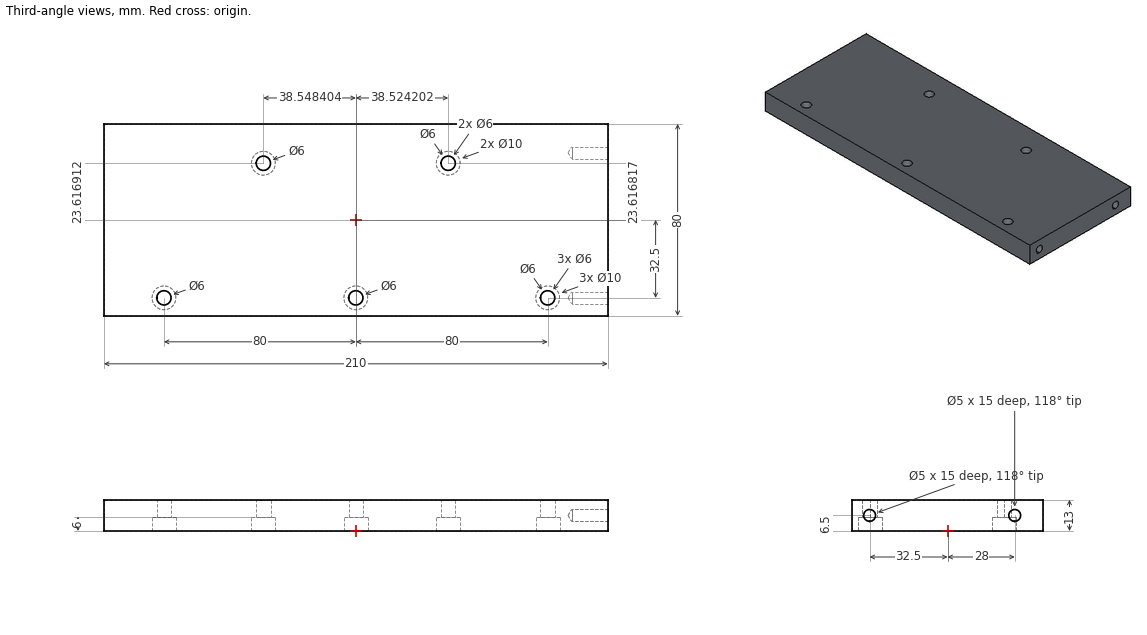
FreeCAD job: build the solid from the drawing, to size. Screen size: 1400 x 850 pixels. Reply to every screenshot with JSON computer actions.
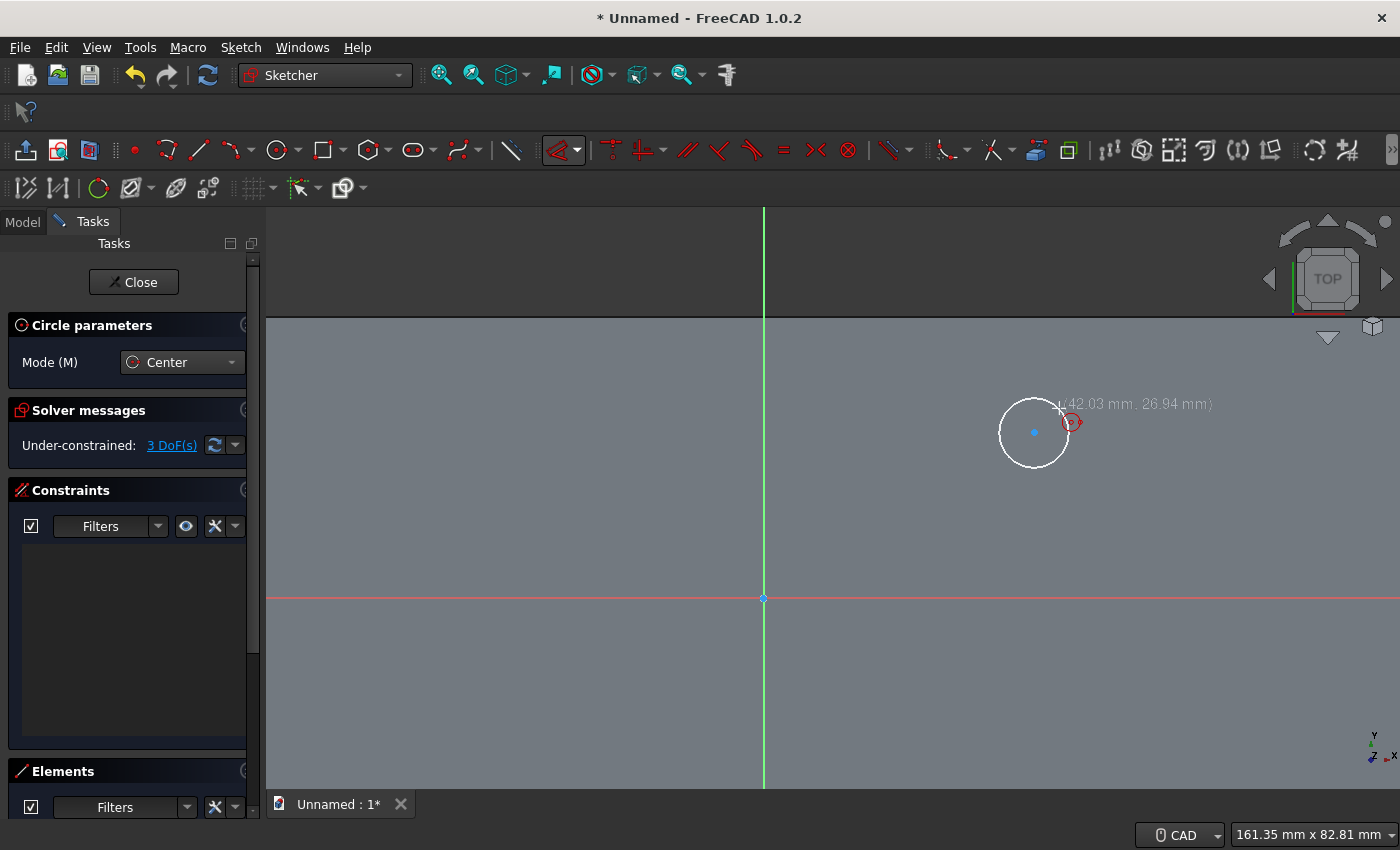
{"action": "left_click", "coordinate": [493, 432]}
{"action": "left_click", "coordinate": [518, 408]}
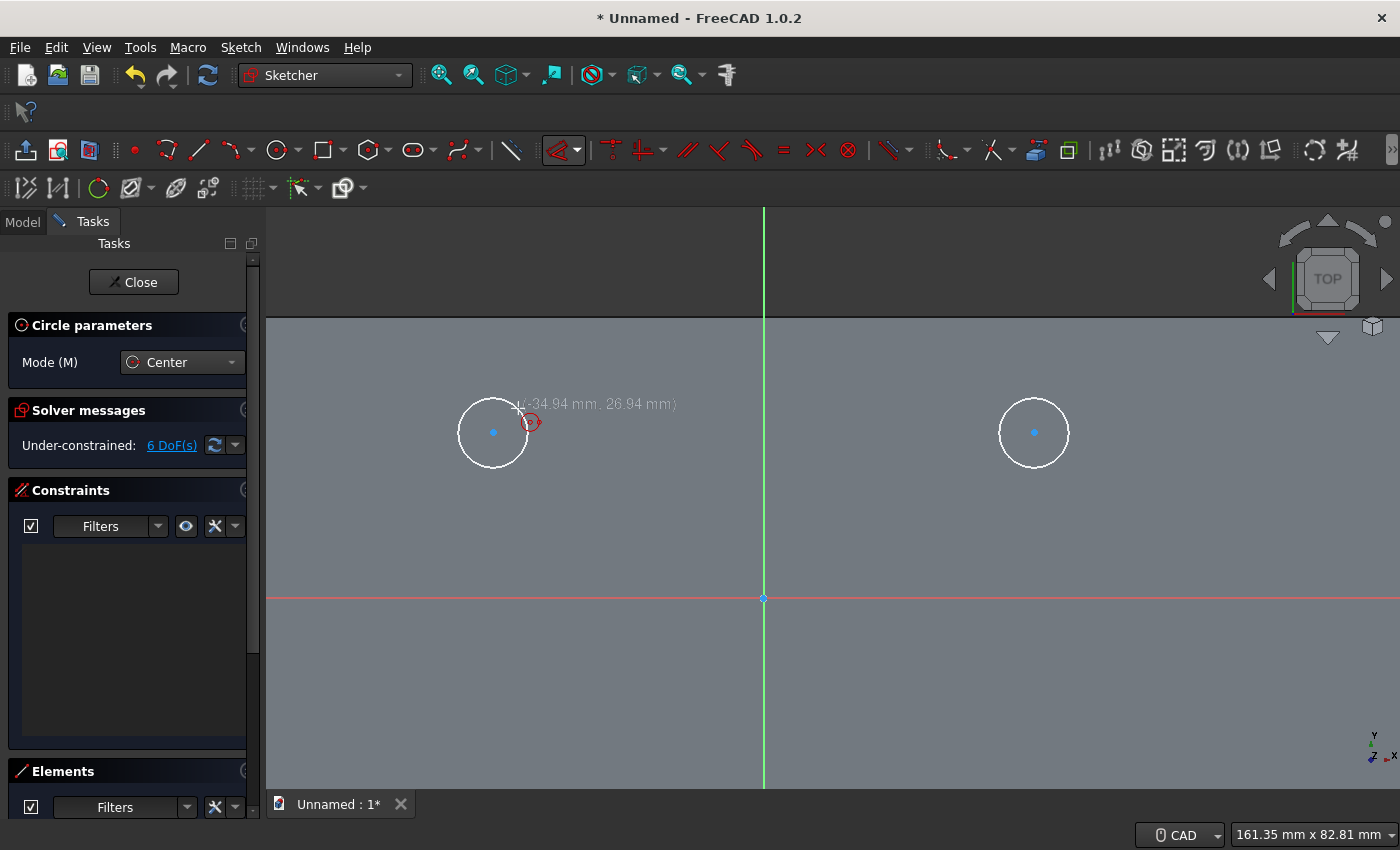
{"action": "left_click", "coordinate": [1034, 433]}
{"action": "left_click", "coordinate": [1049, 417]}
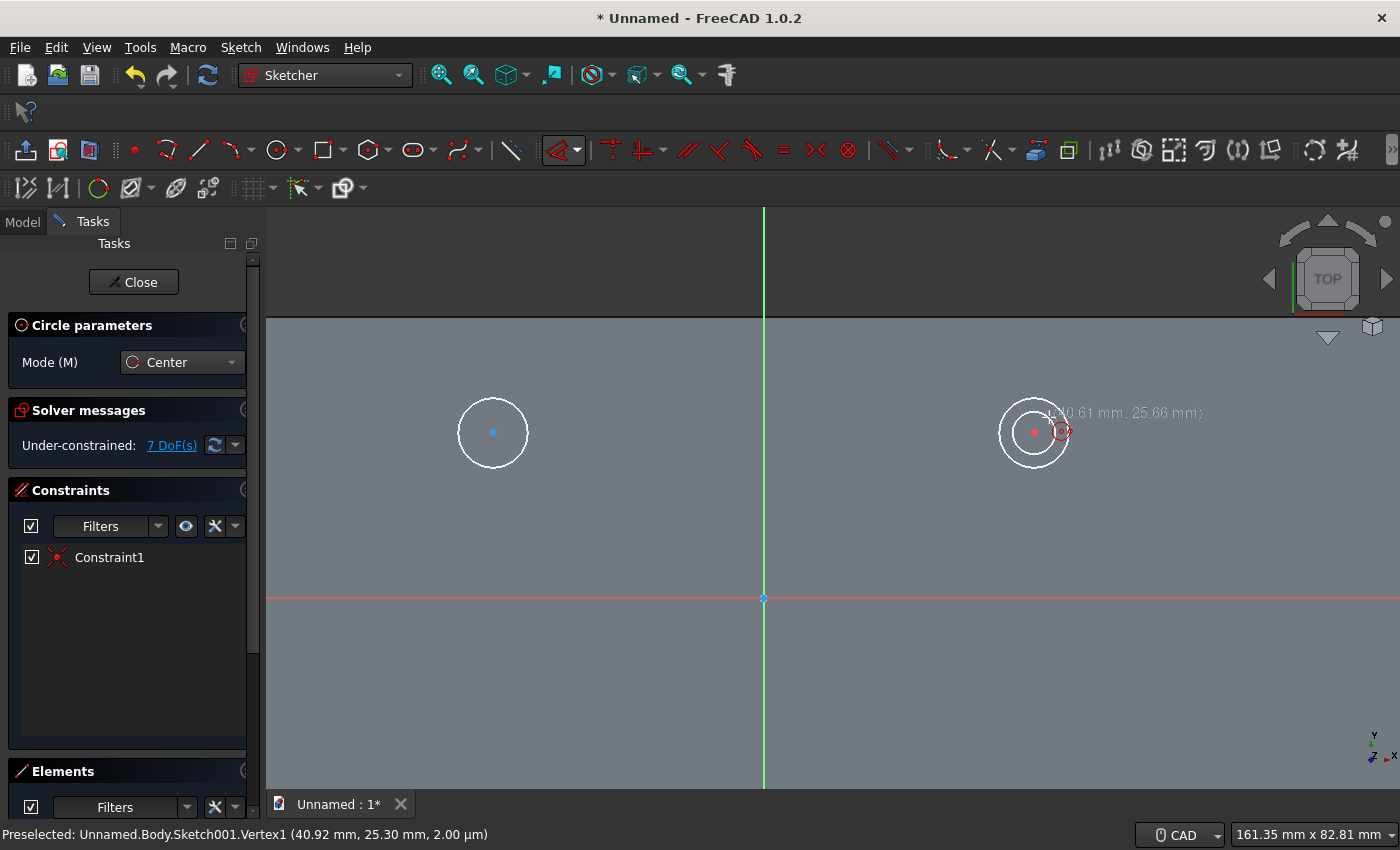
{"action": "left_click", "coordinate": [493, 433]}
{"action": "left_click", "coordinate": [508, 417]}
{"action": "key", "text": "Escape"}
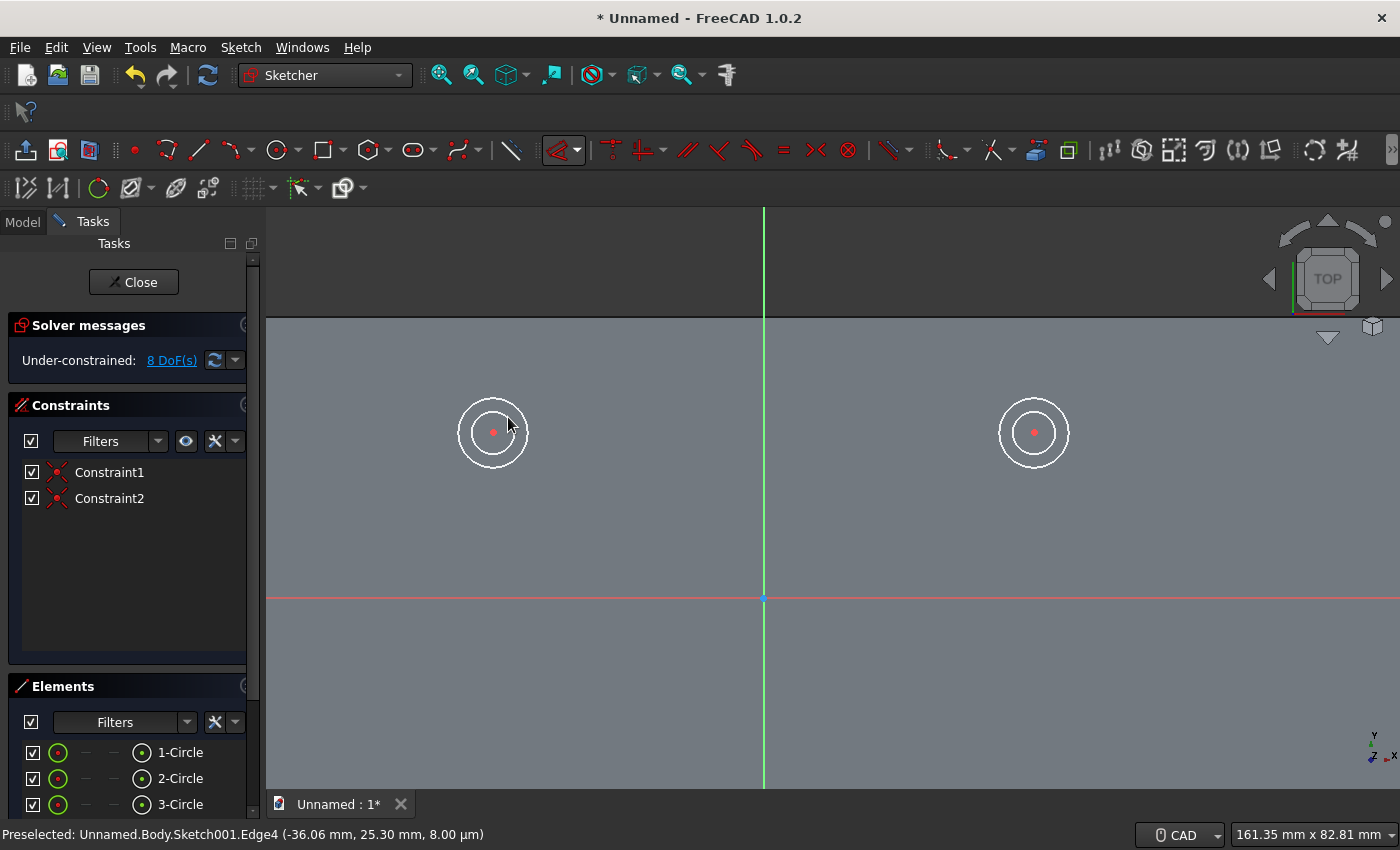
{"action": "left_click", "coordinate": [1058, 408]}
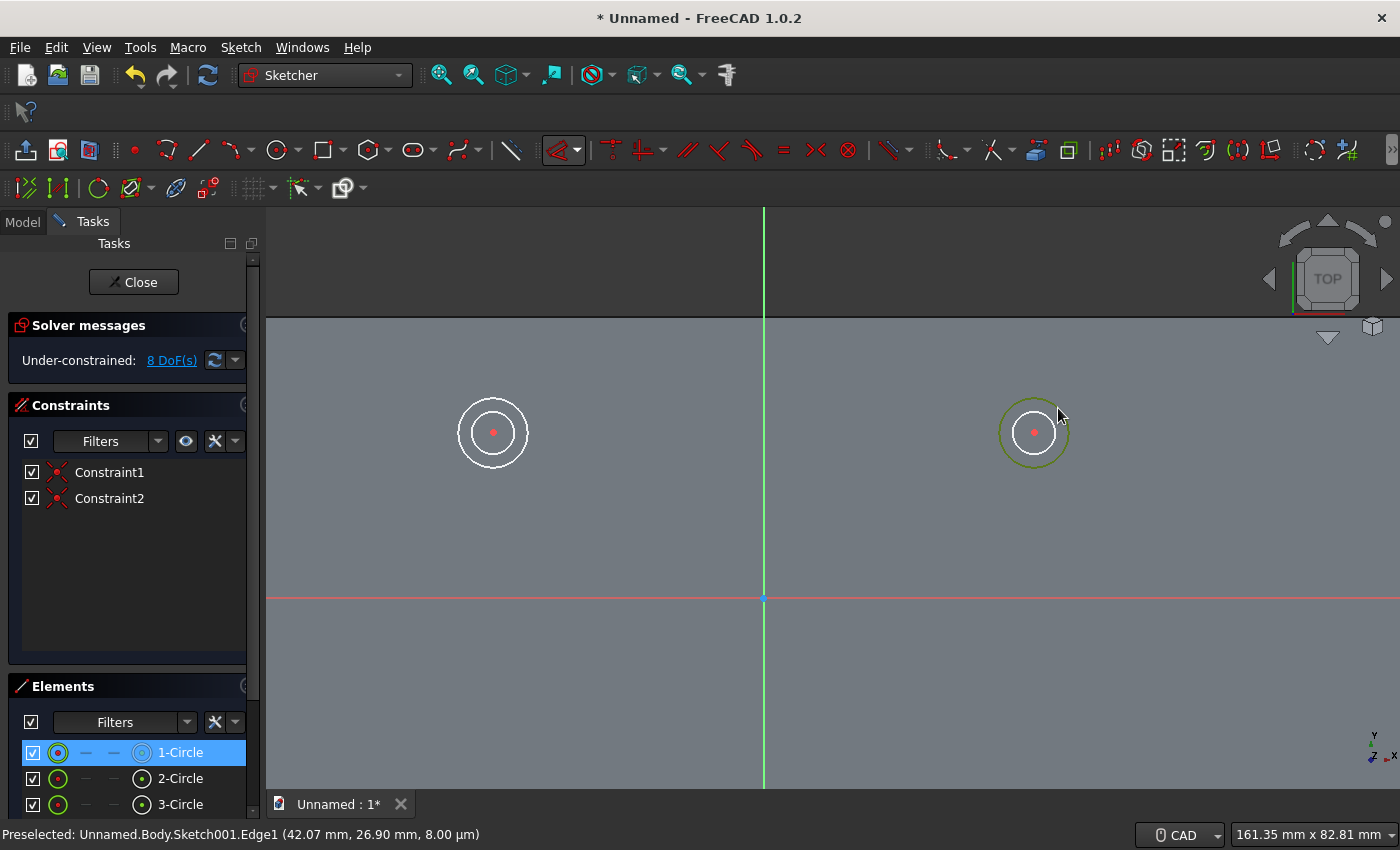
{"action": "left_click", "coordinate": [517, 408]}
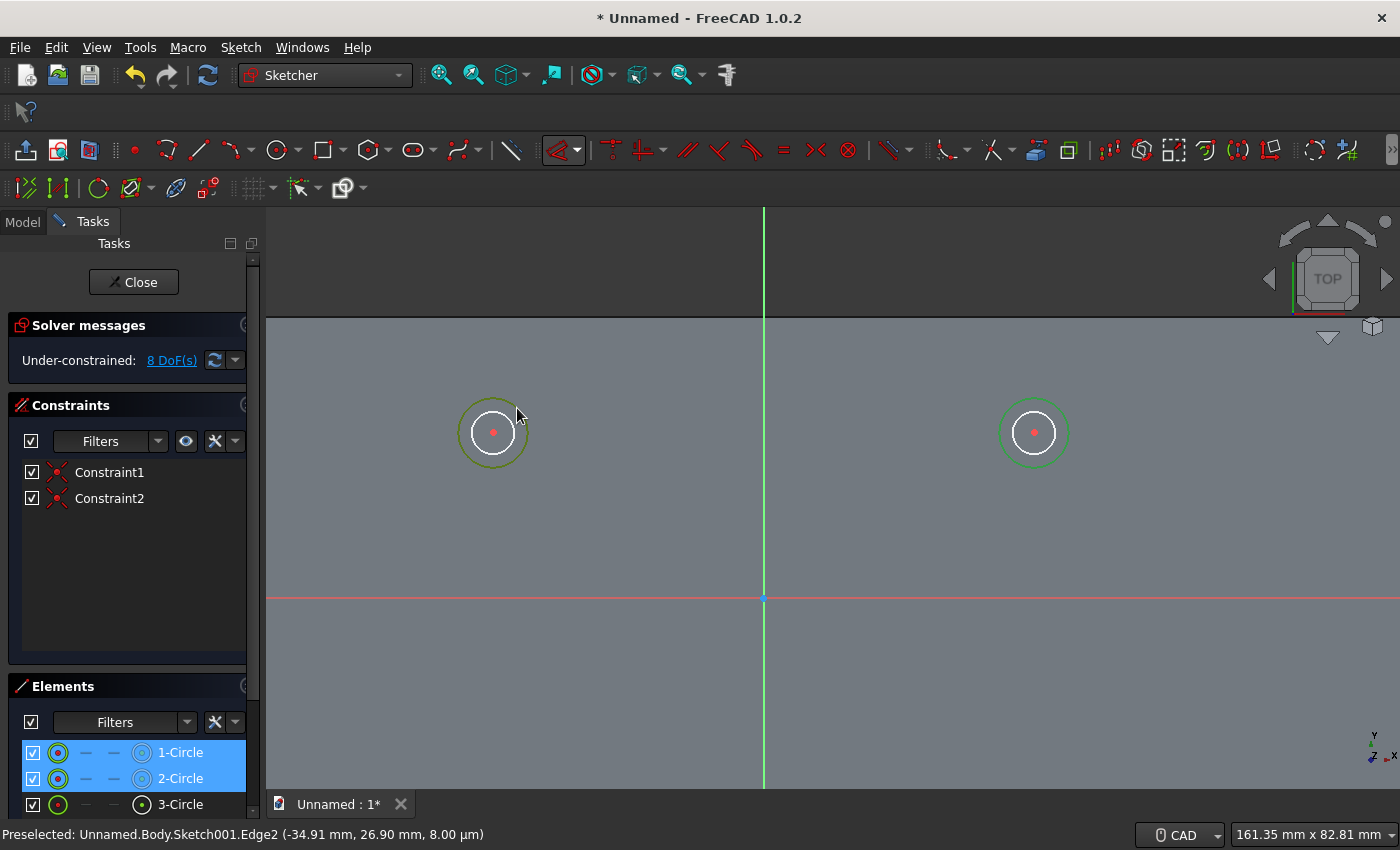
{"action": "left_click", "coordinate": [784, 150]}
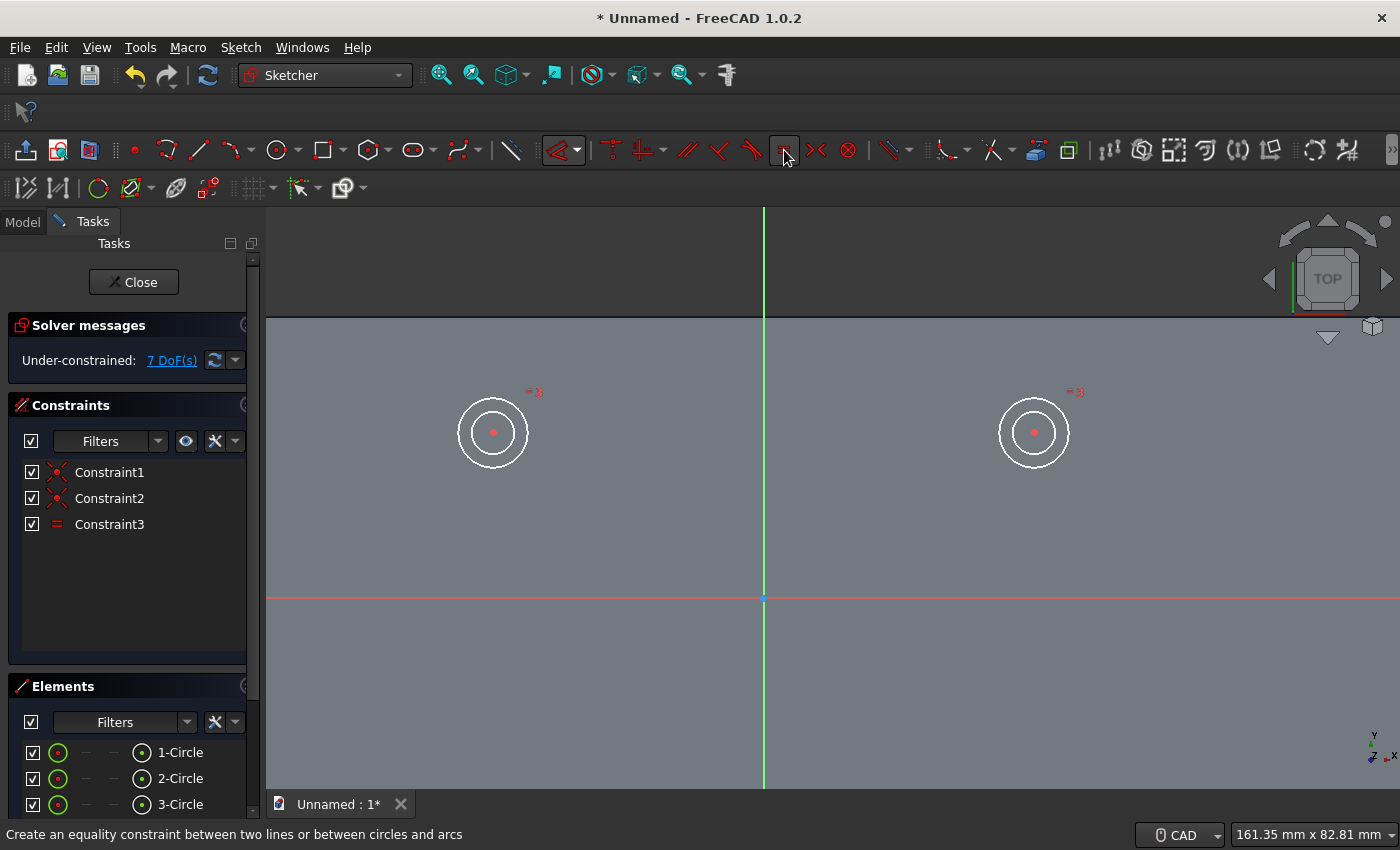
{"action": "left_click", "coordinate": [1049, 418]}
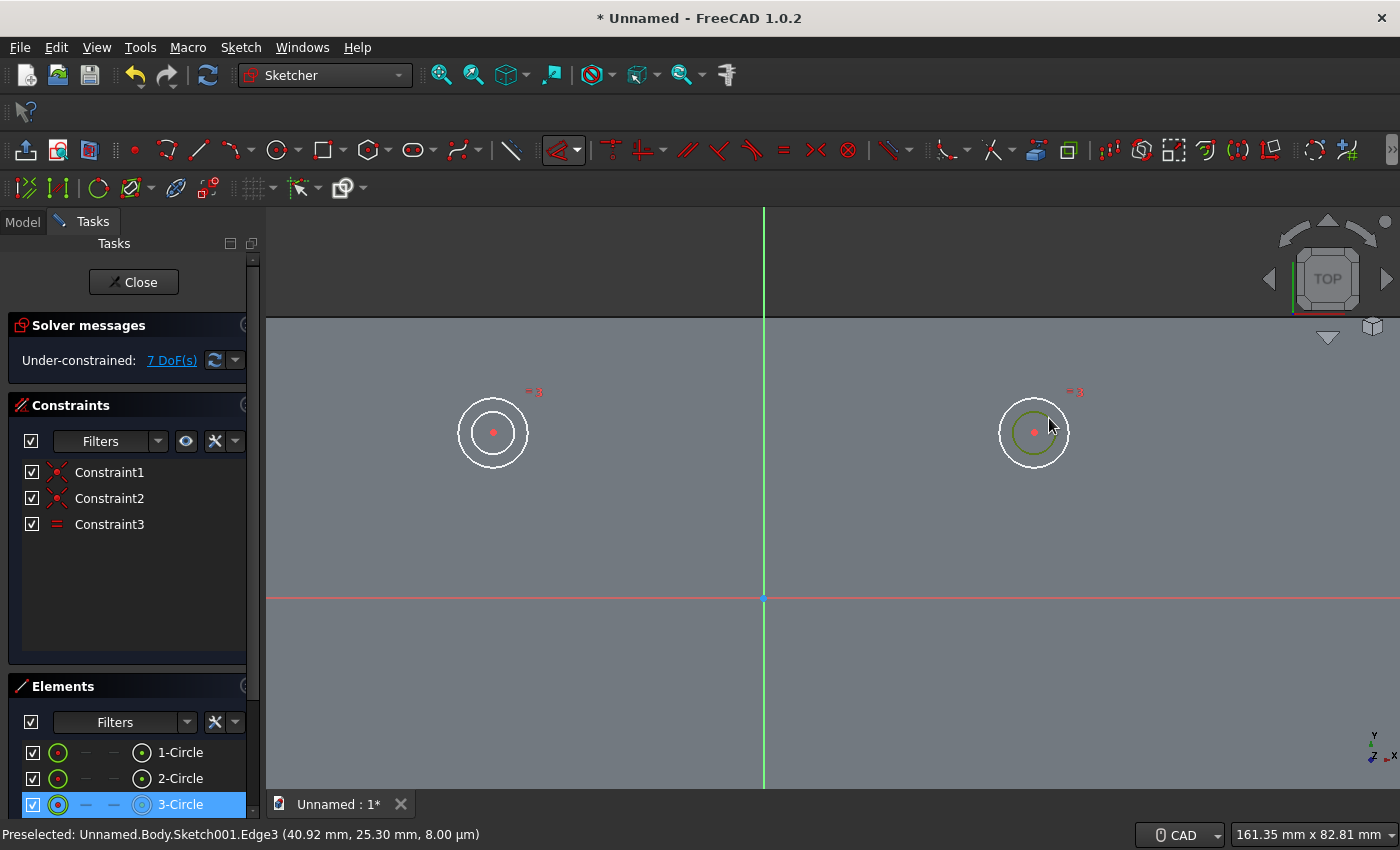
{"action": "left_click", "coordinate": [508, 418]}